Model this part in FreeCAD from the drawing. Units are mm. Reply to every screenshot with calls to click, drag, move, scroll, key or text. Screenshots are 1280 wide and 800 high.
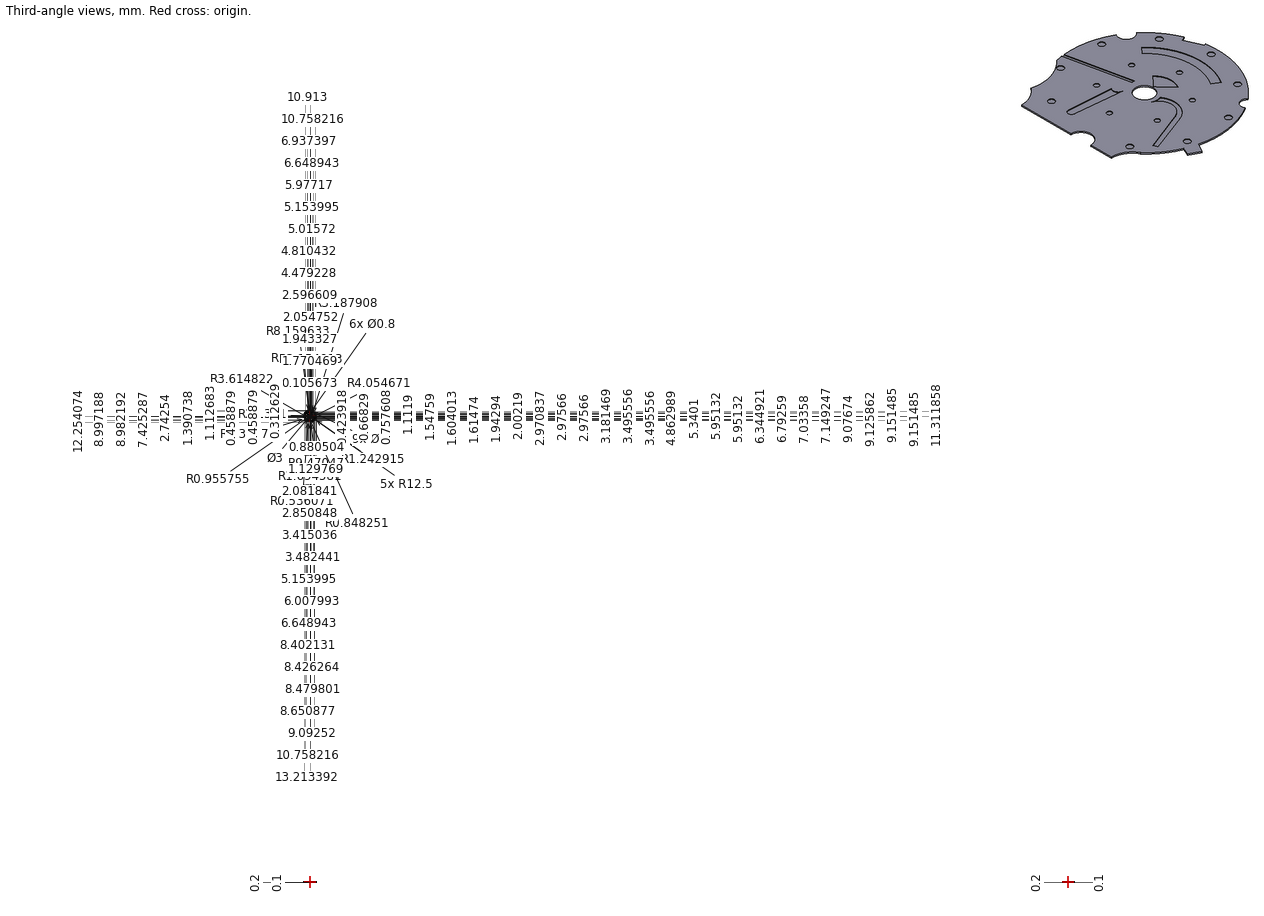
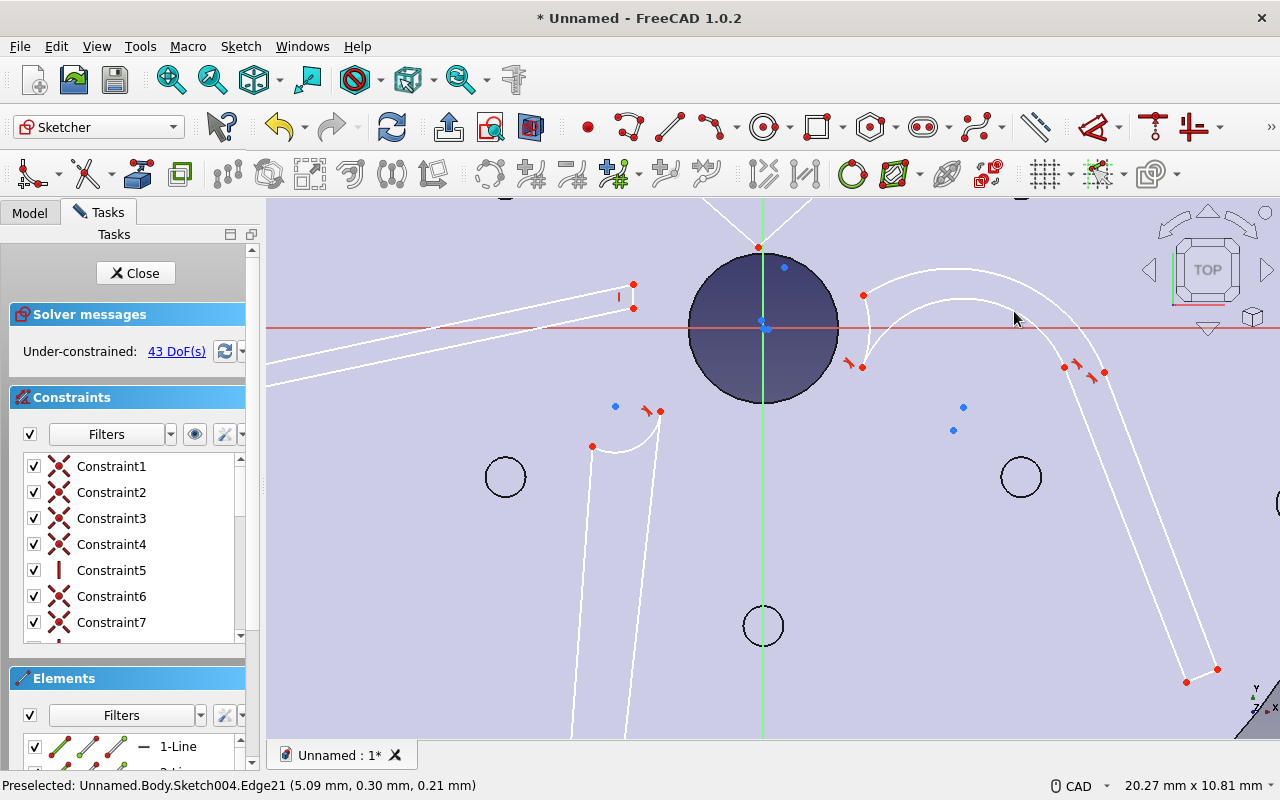
scroll(730, 547, down, 5)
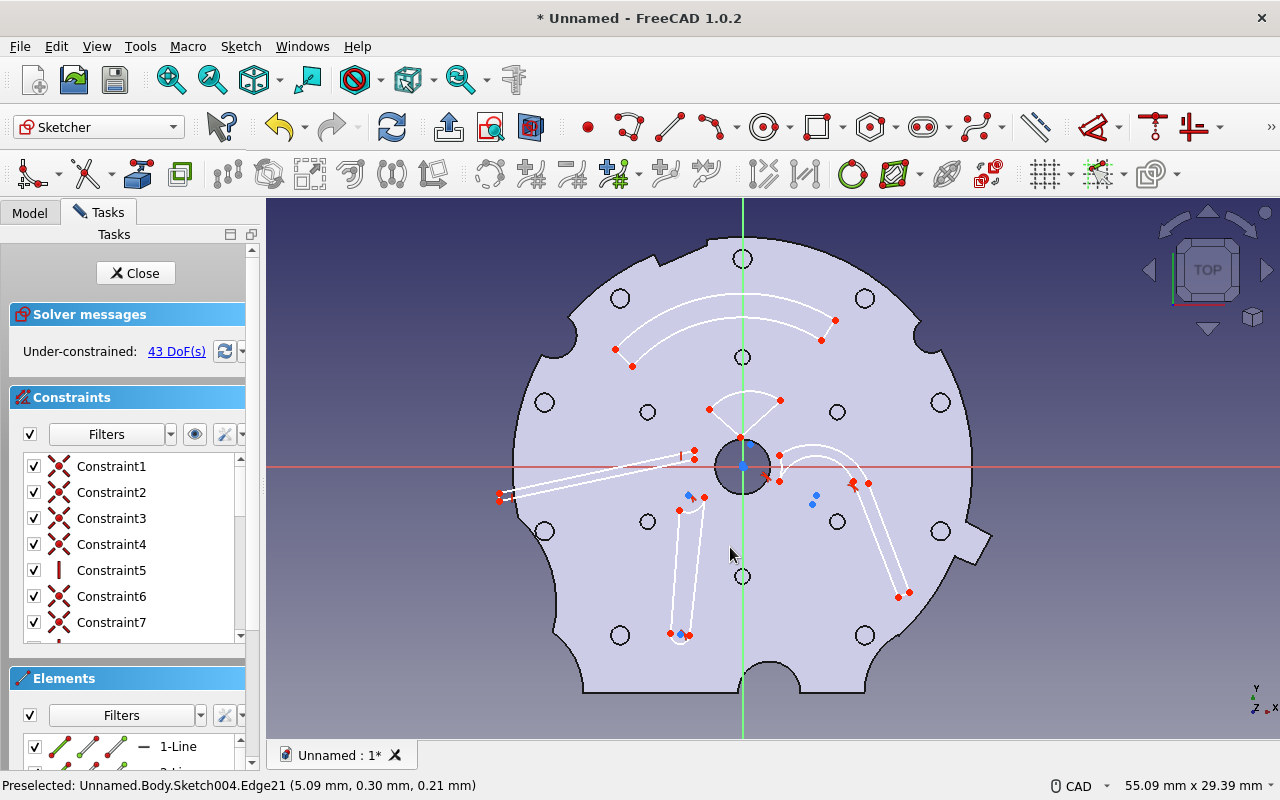
click(764, 319)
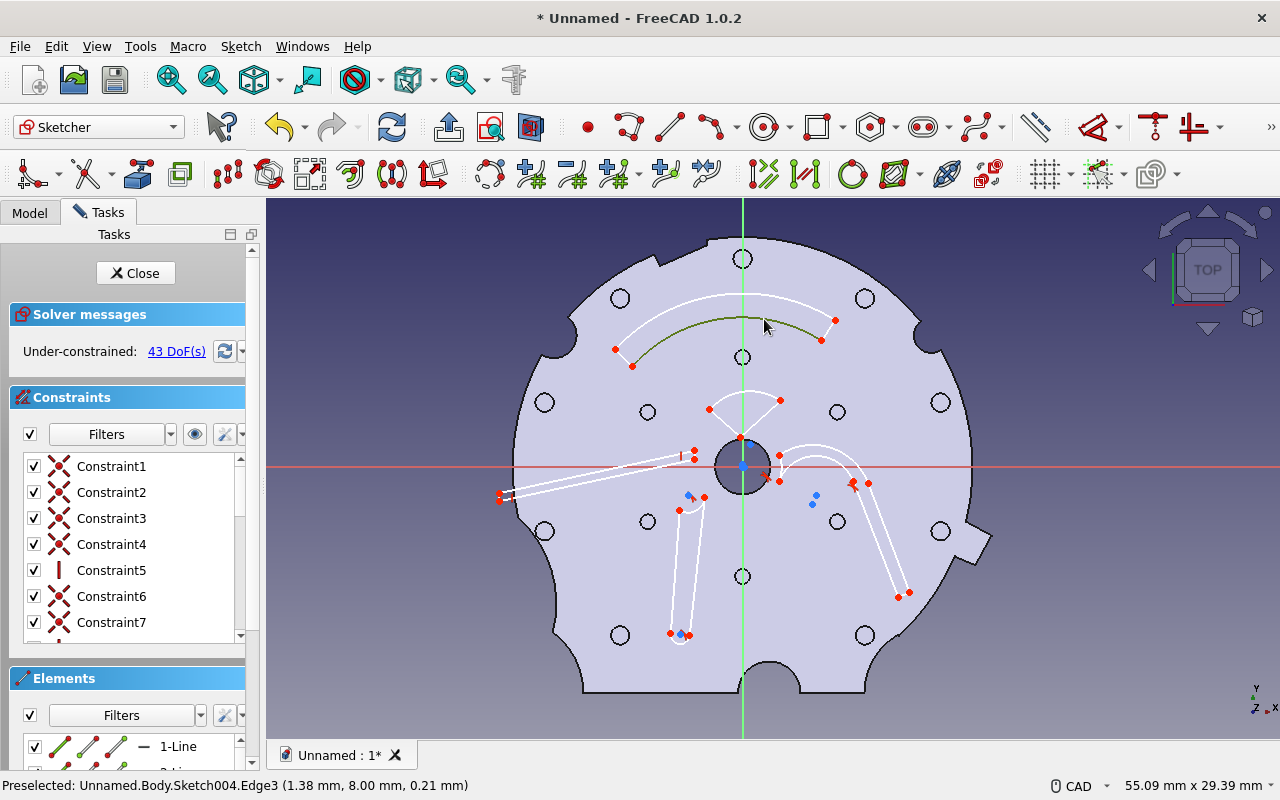
click(768, 295)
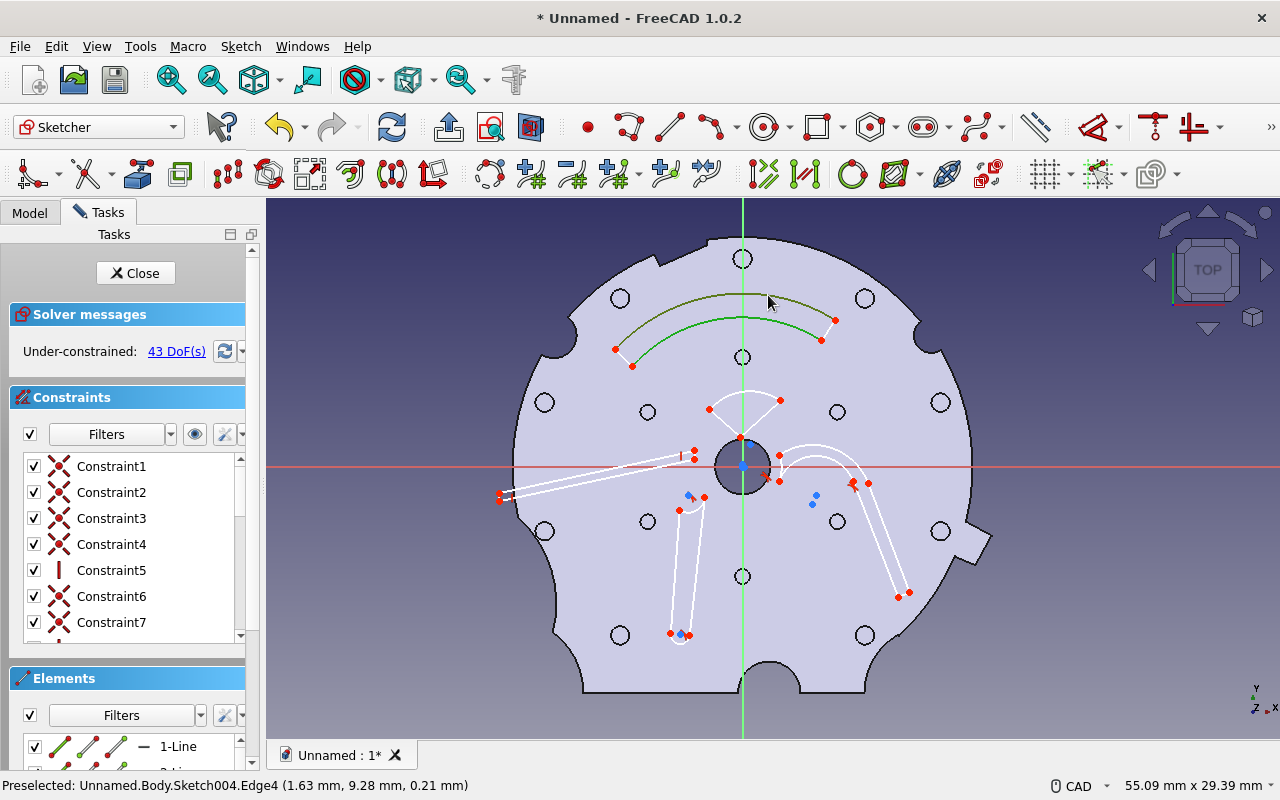
key(c)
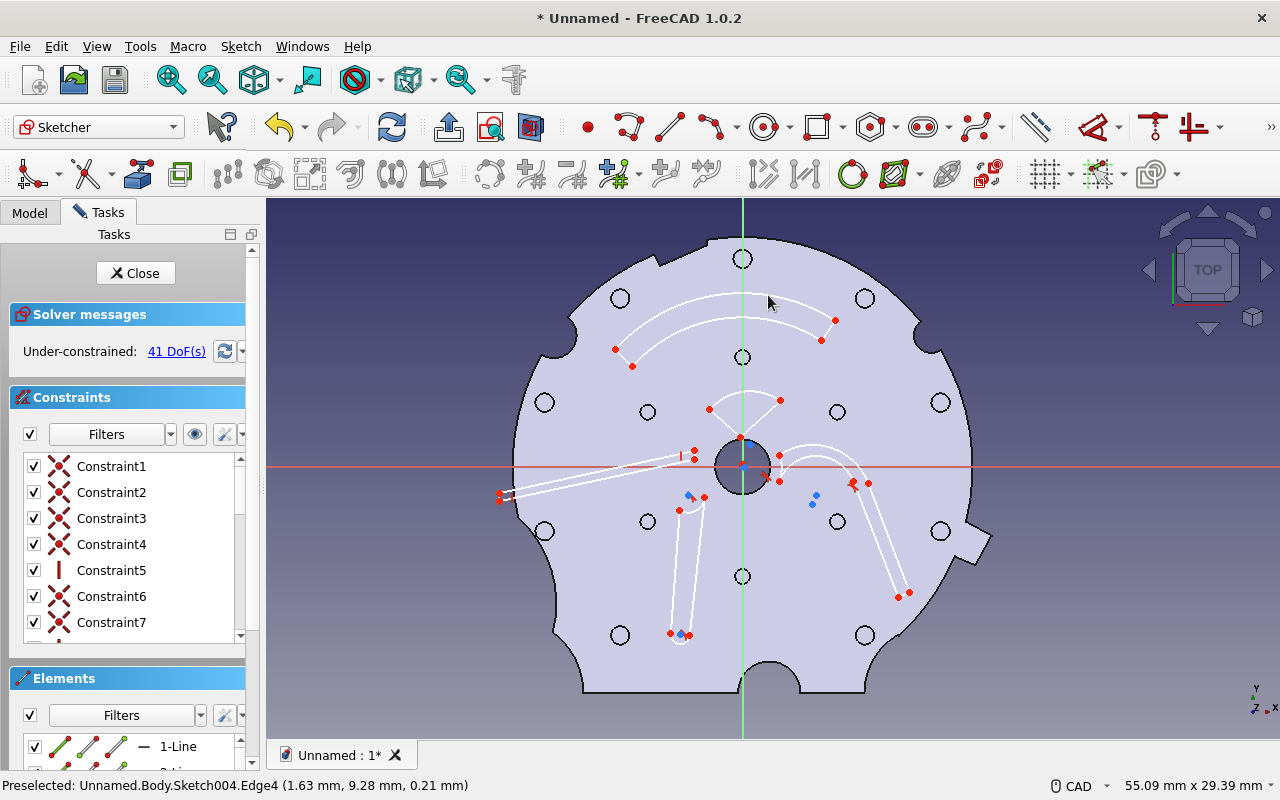
click(764, 319)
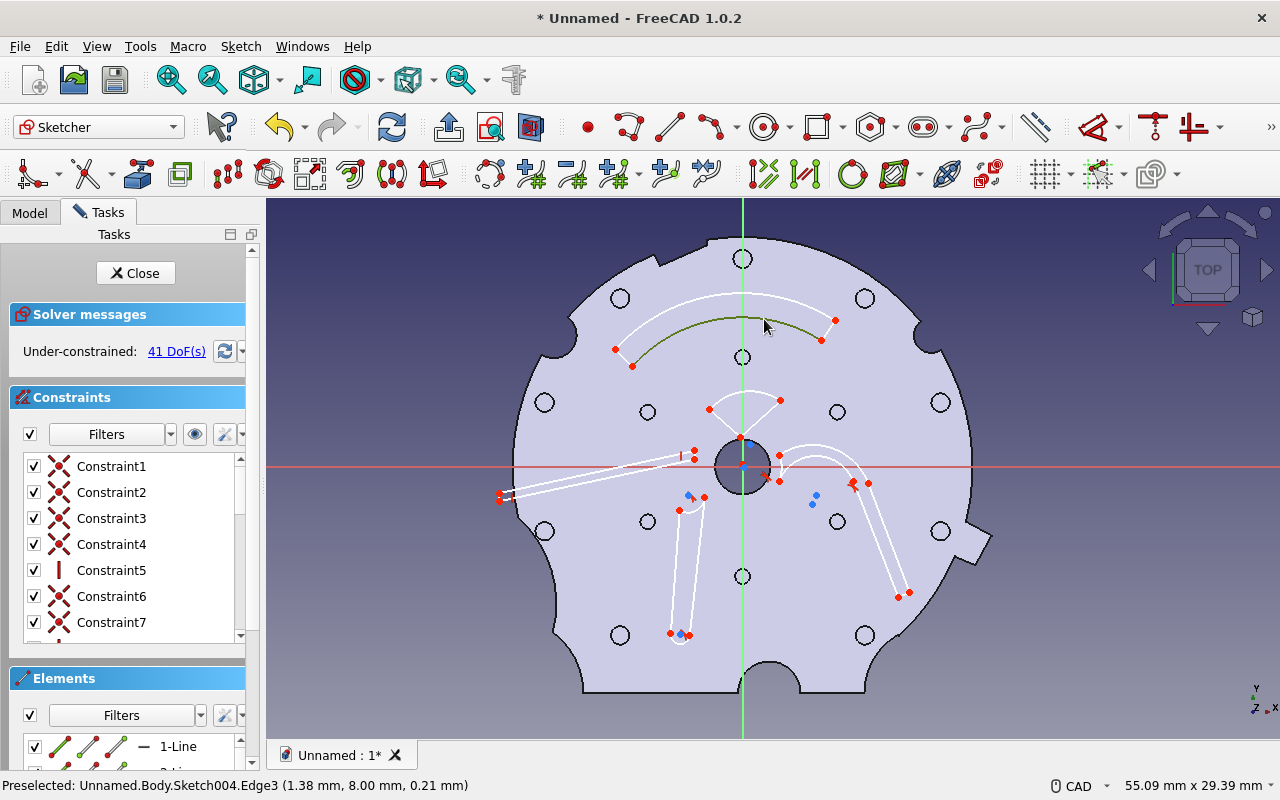
scroll(781, 460, up, 5)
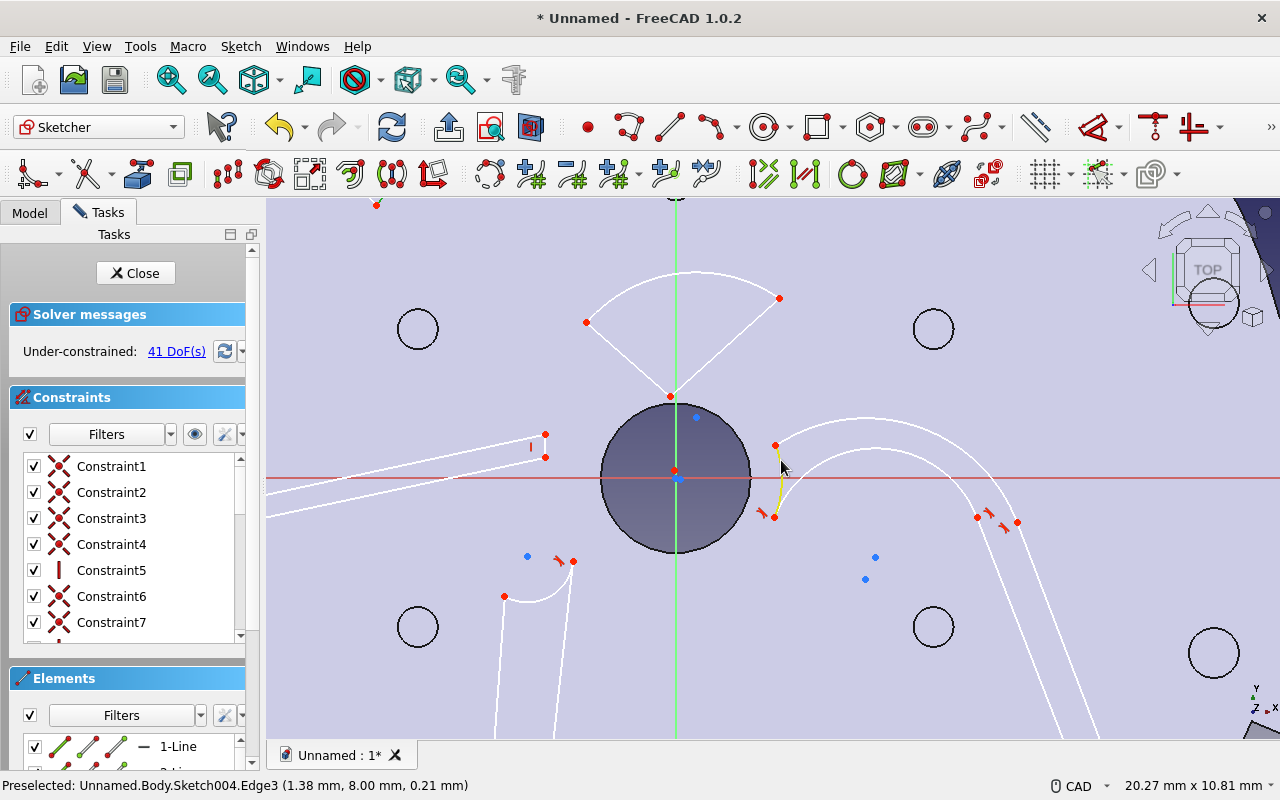
click(780, 460)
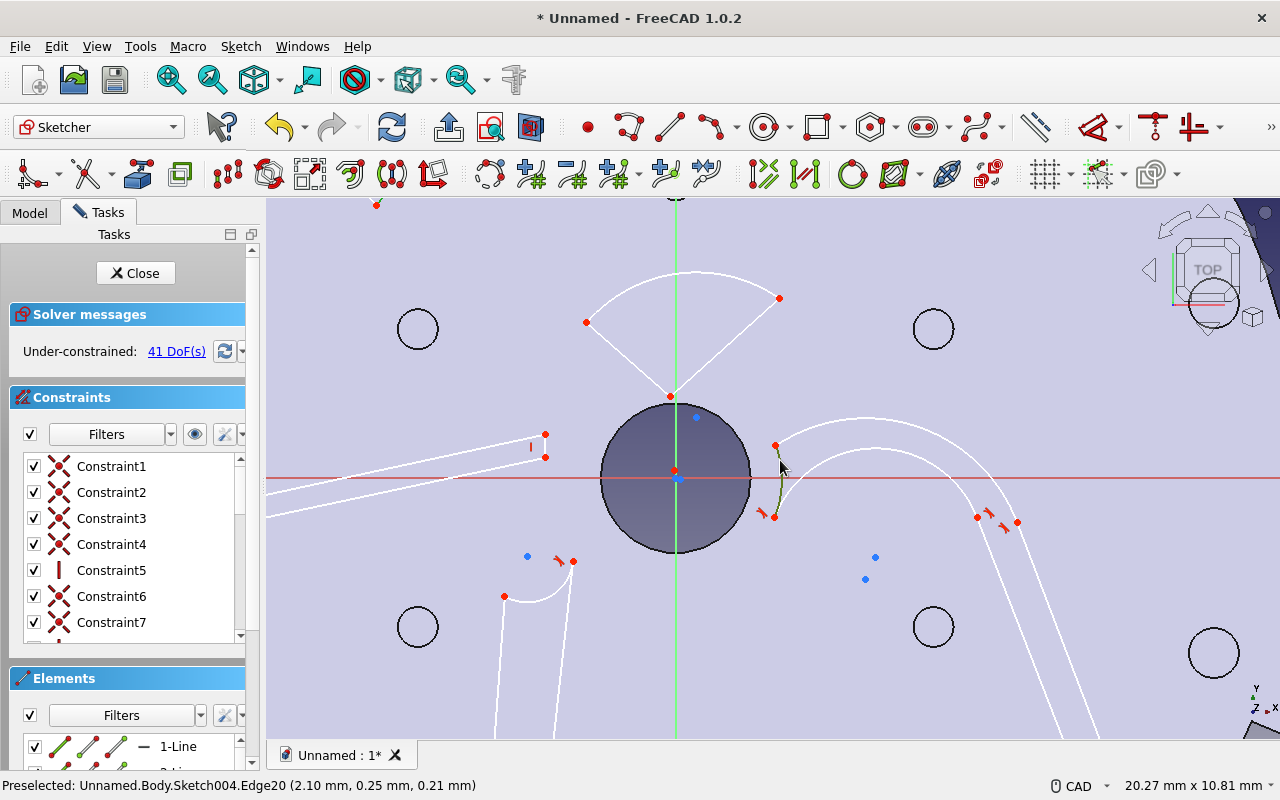
click(1153, 128)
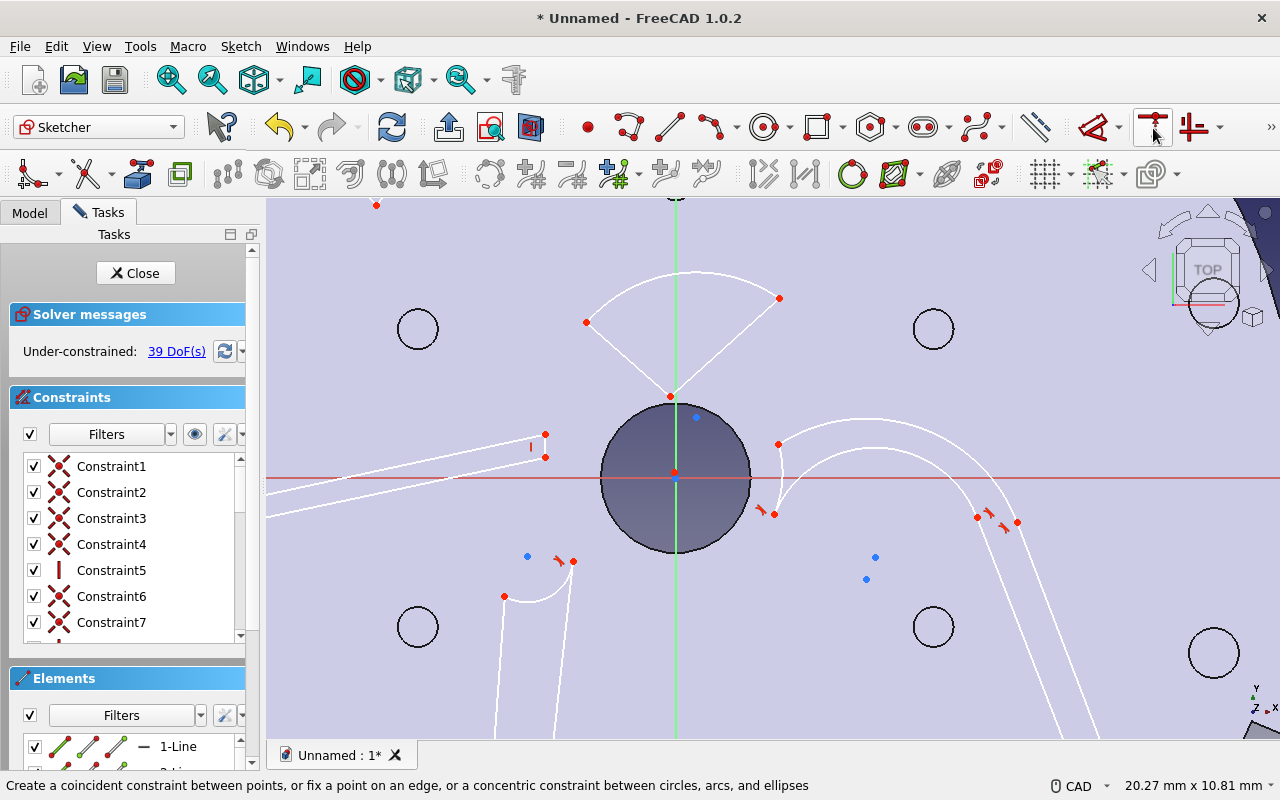
scroll(675, 475, up, 3)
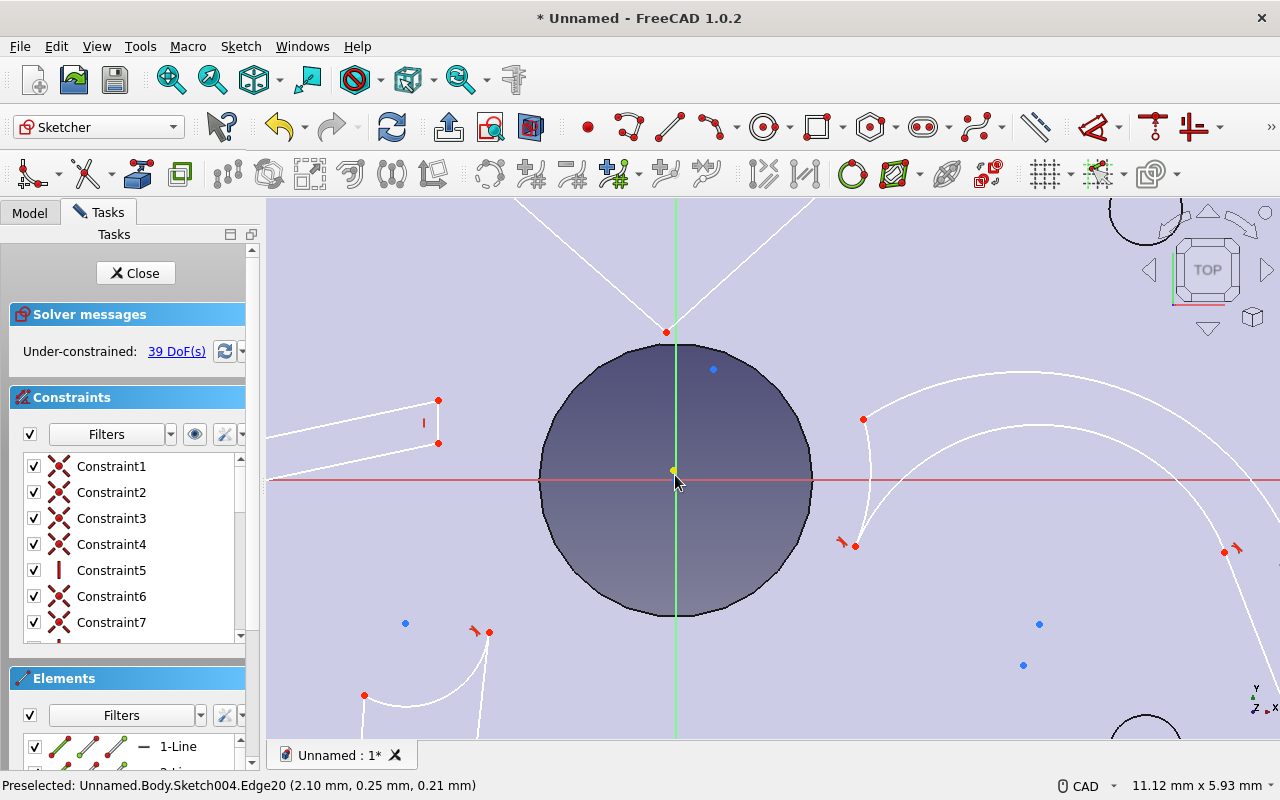
drag(664, 461, 686, 490)